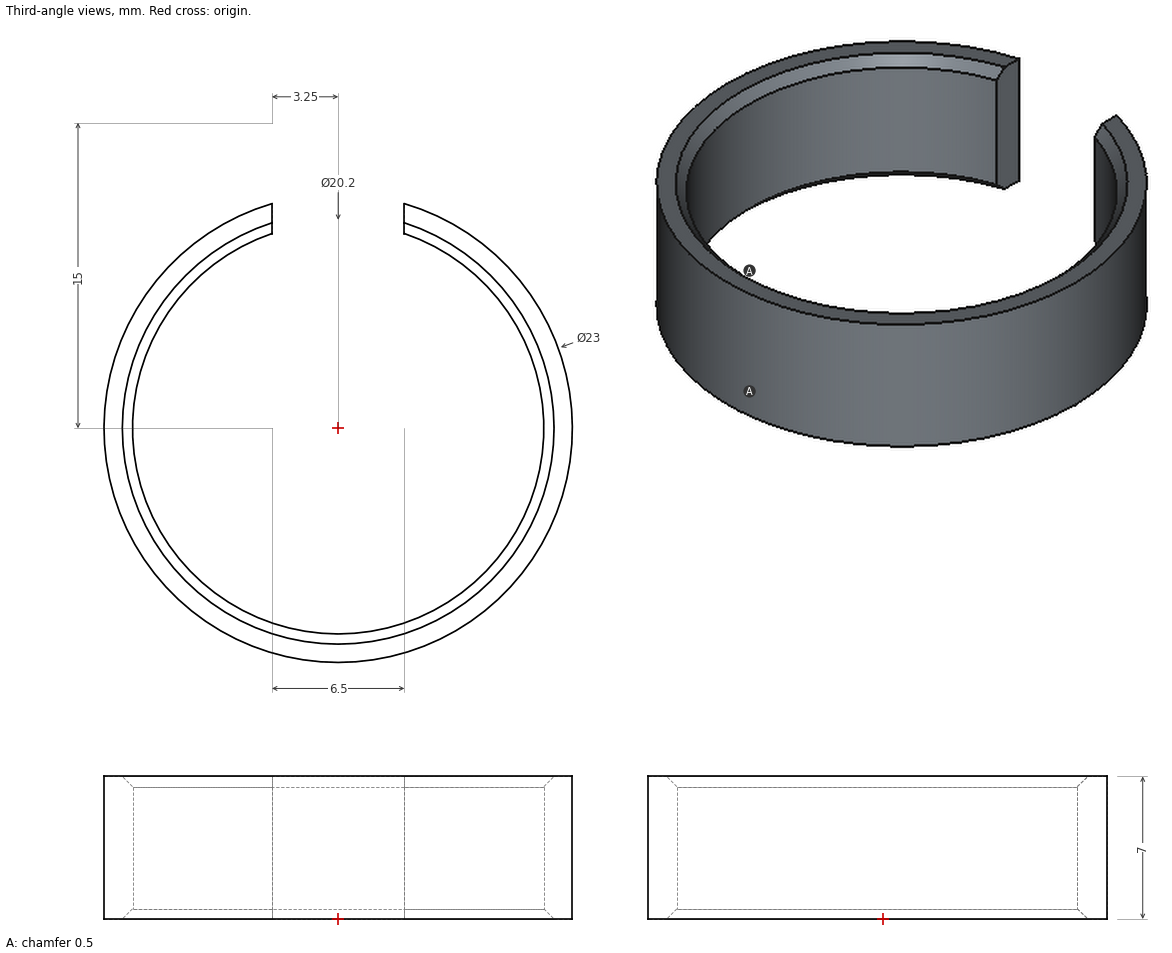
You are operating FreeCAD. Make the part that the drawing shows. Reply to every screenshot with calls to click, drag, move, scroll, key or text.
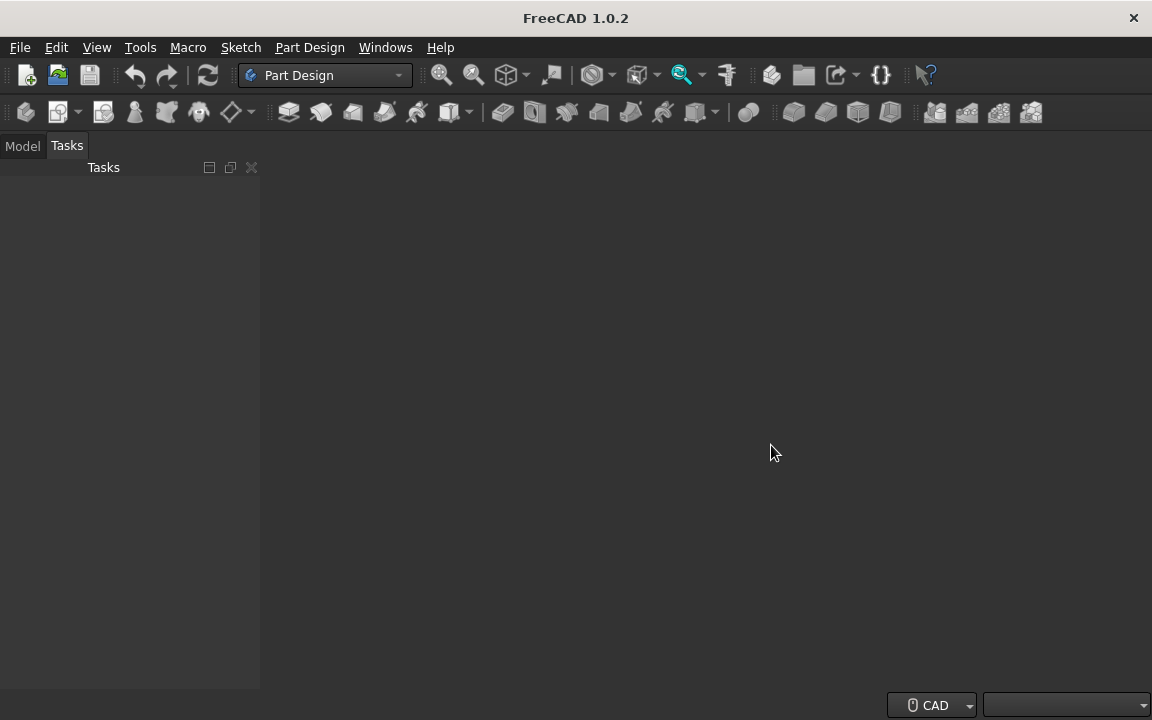
click(26, 76)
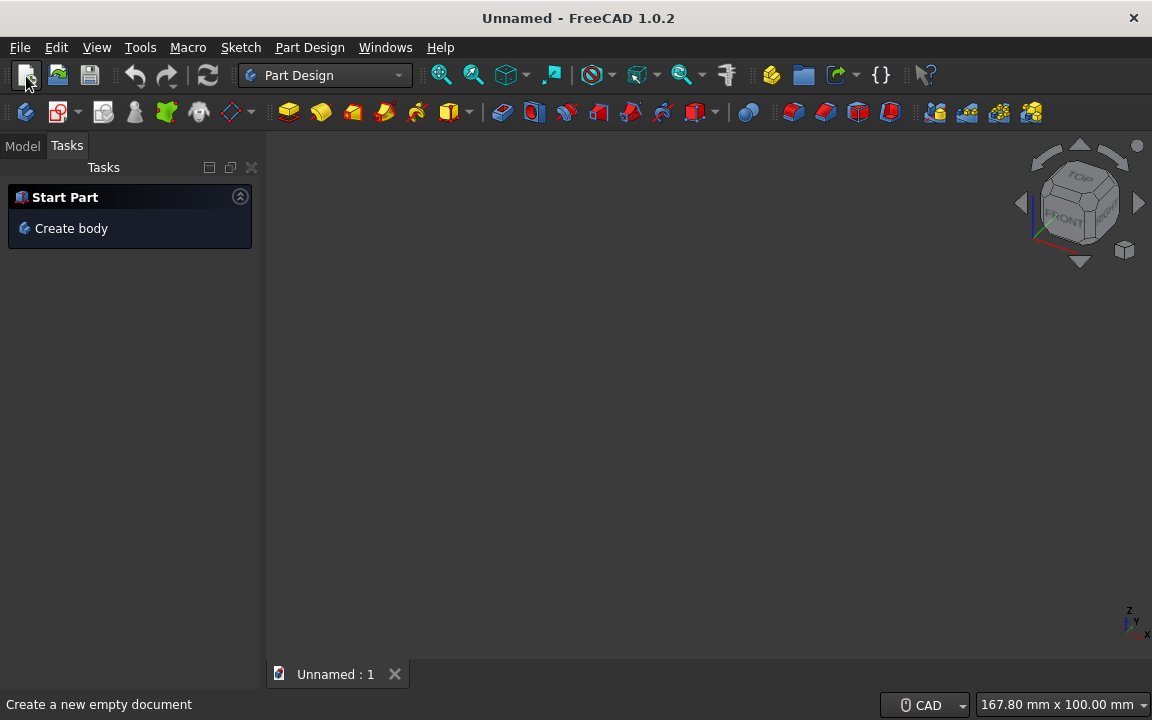
click(58, 112)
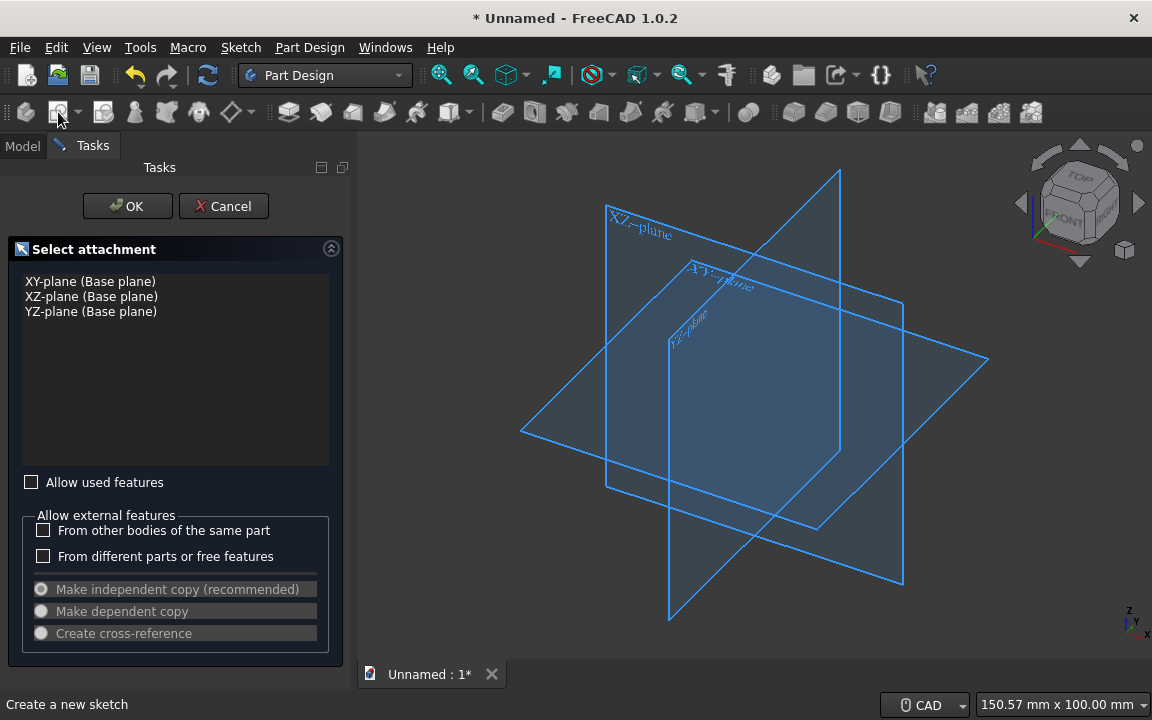
click(82, 282)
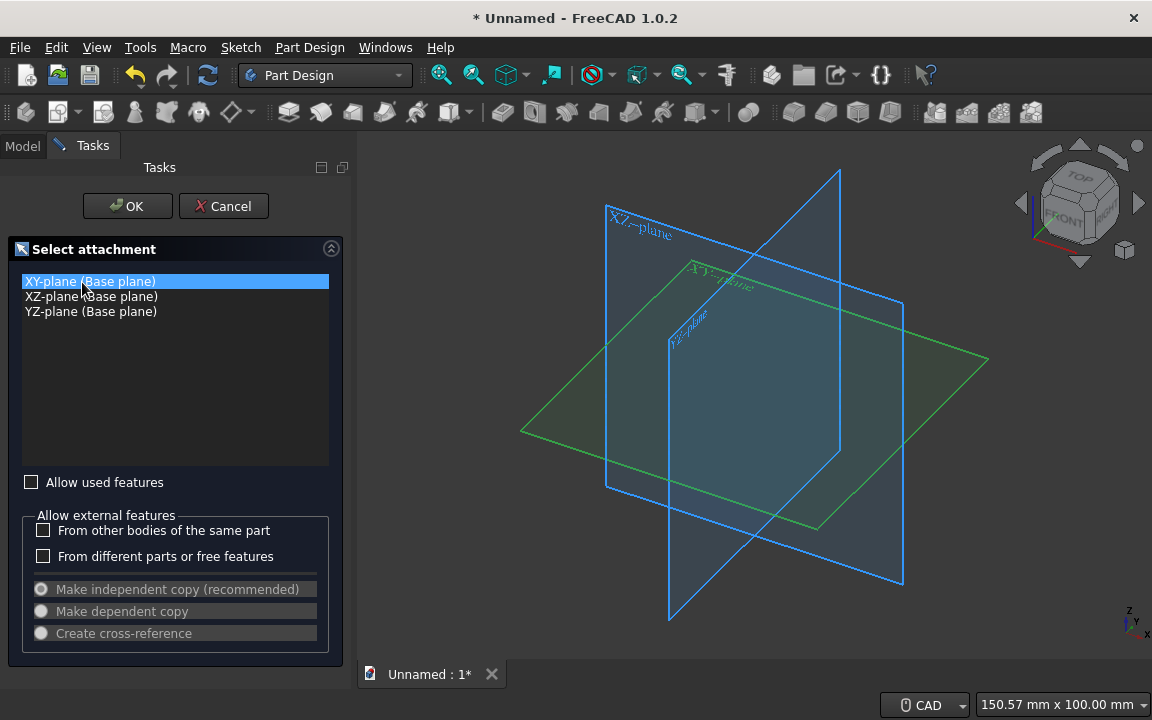
click(128, 206)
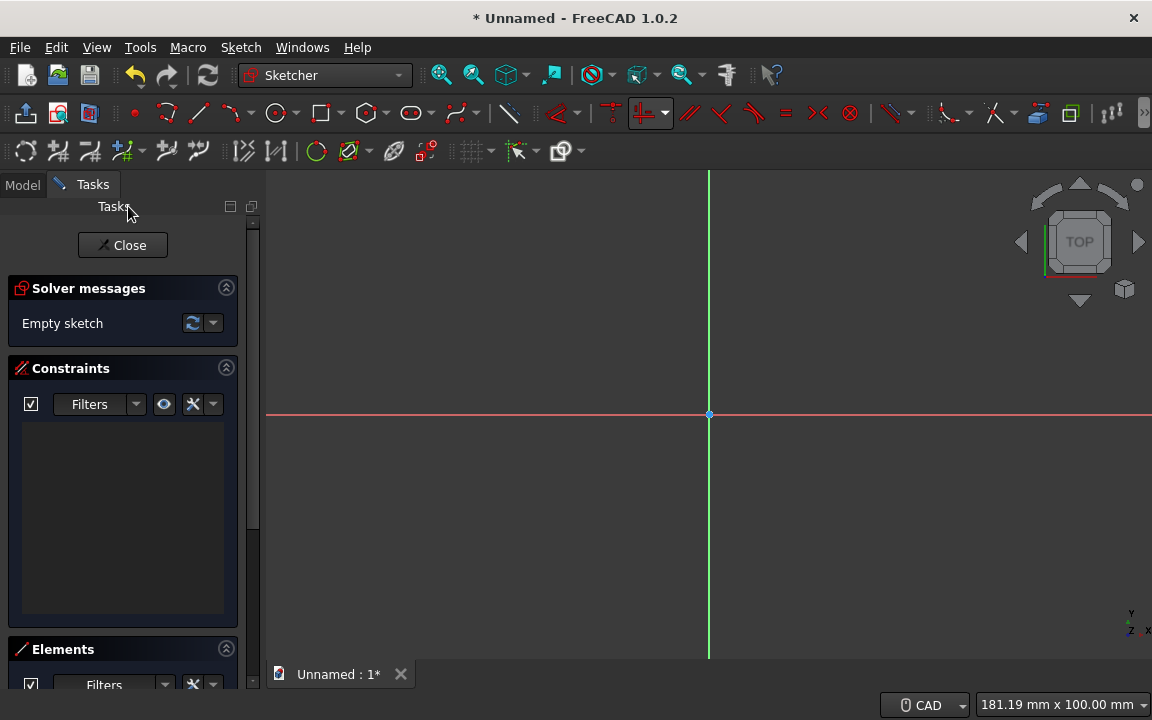
scroll(749, 415, up, 5)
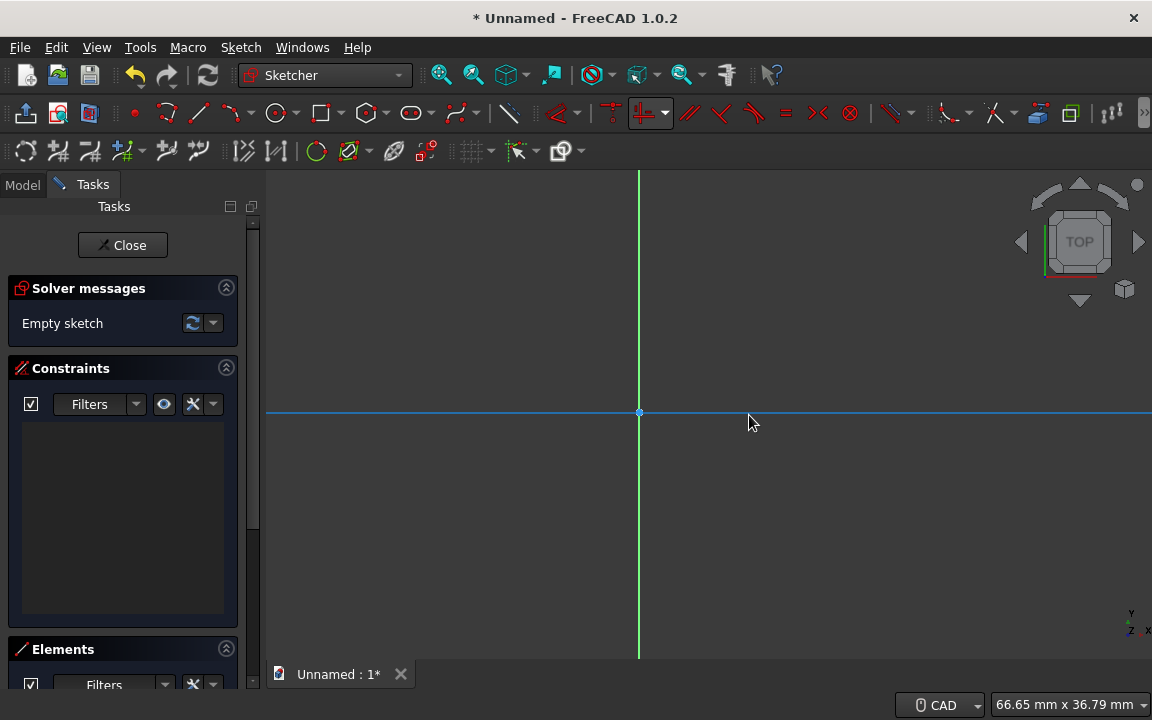
click(276, 114)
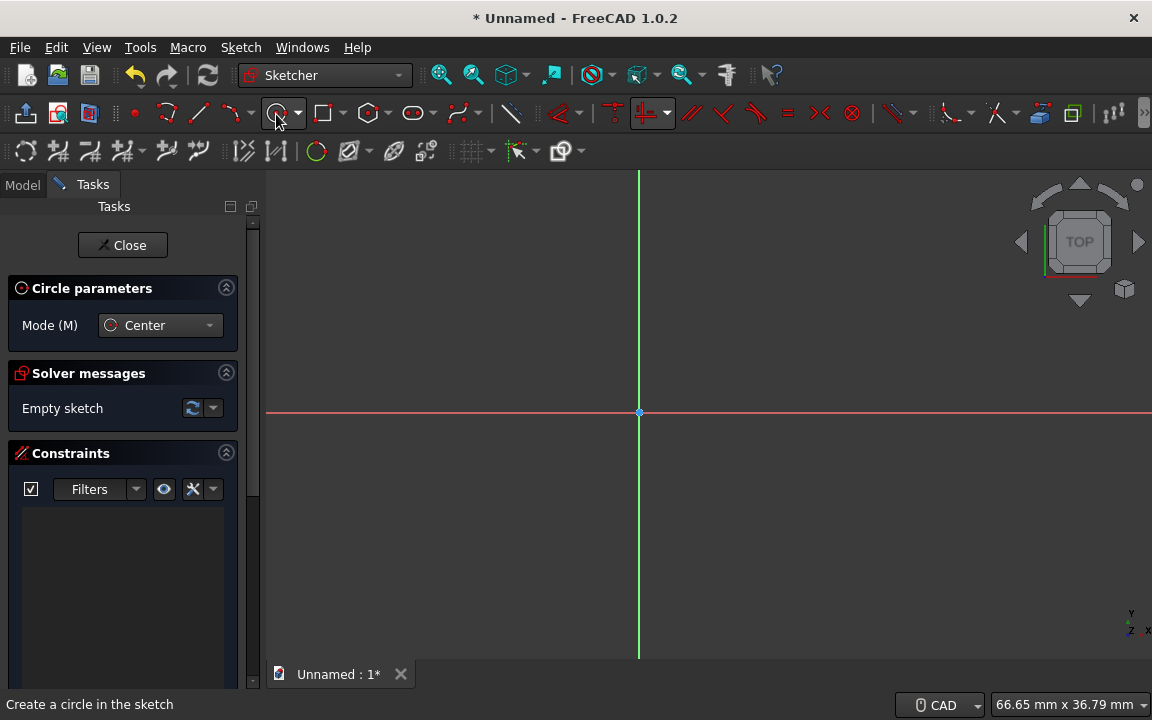
click(639, 413)
click(747, 305)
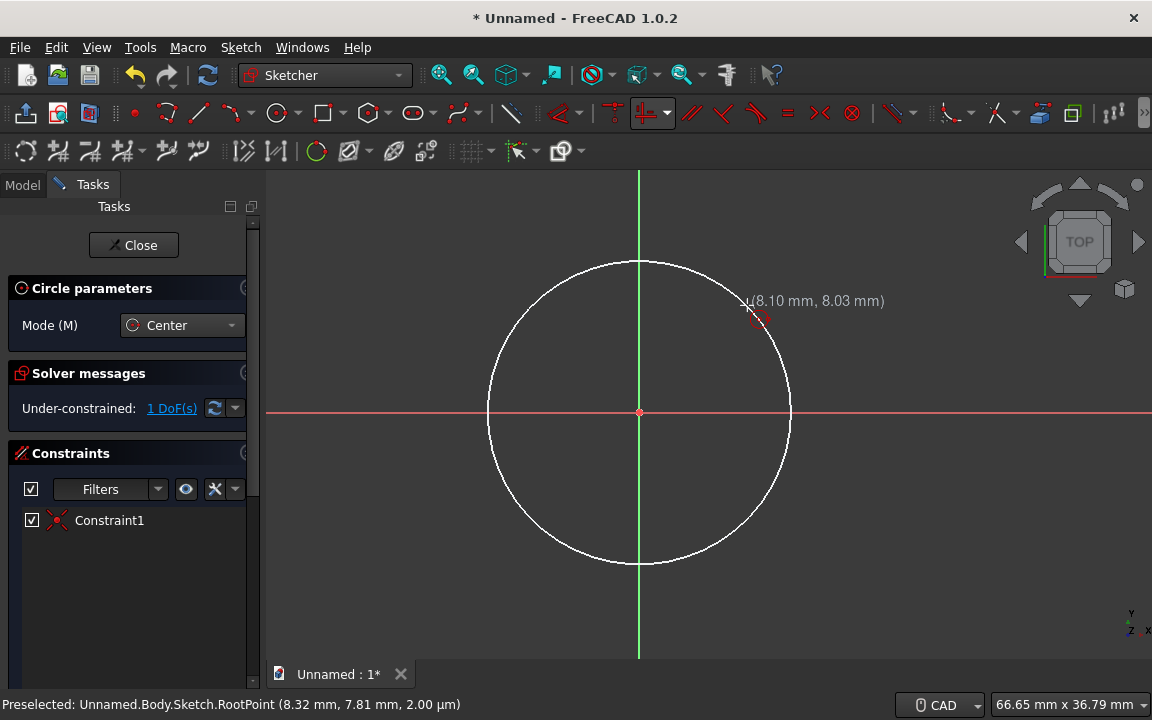
click(639, 413)
click(734, 318)
key(Escape)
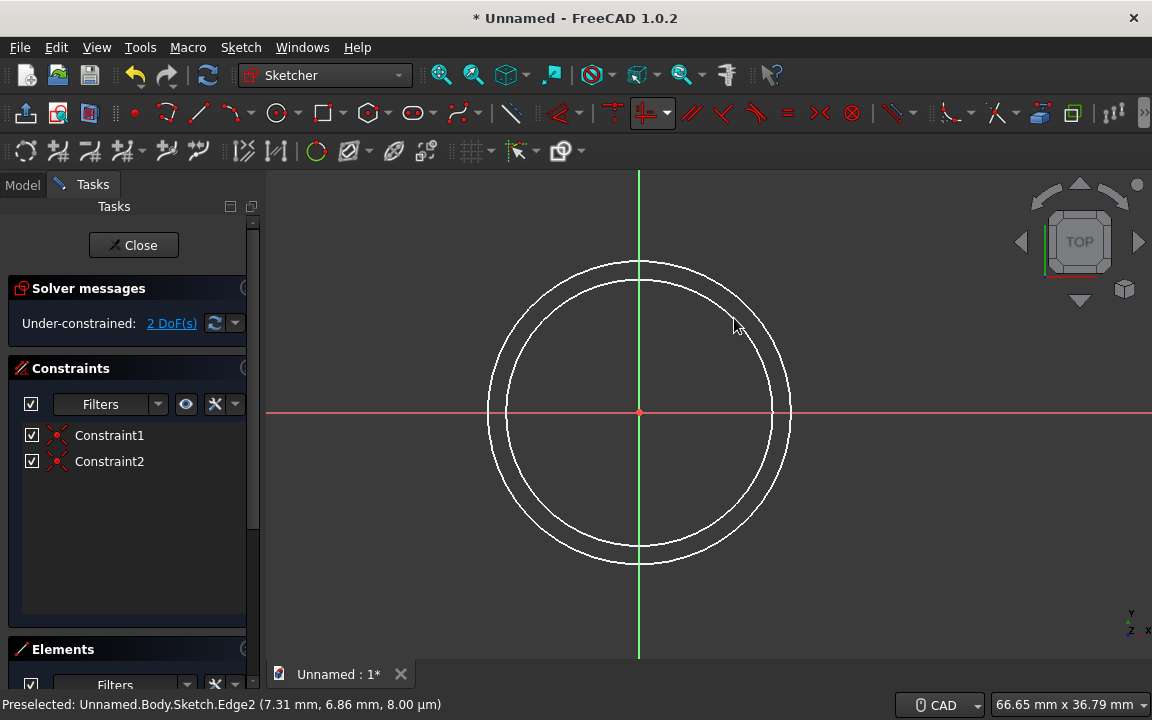
click(558, 114)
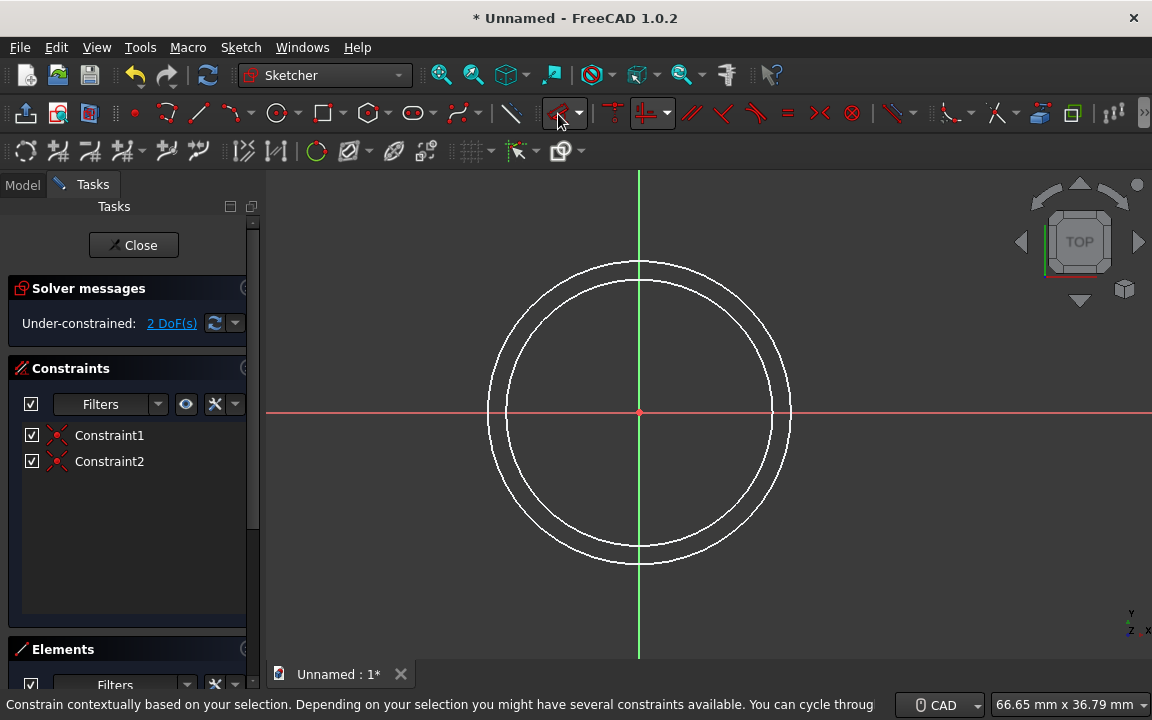
click(746, 305)
click(769, 282)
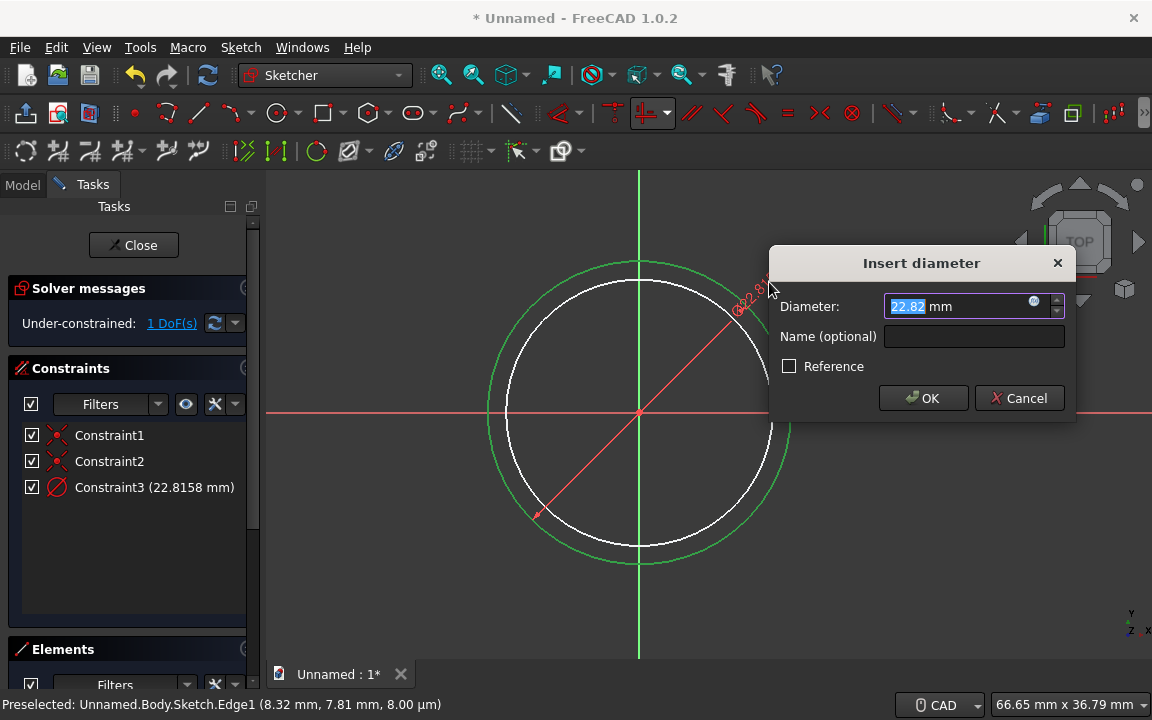
text(23)
key(Return)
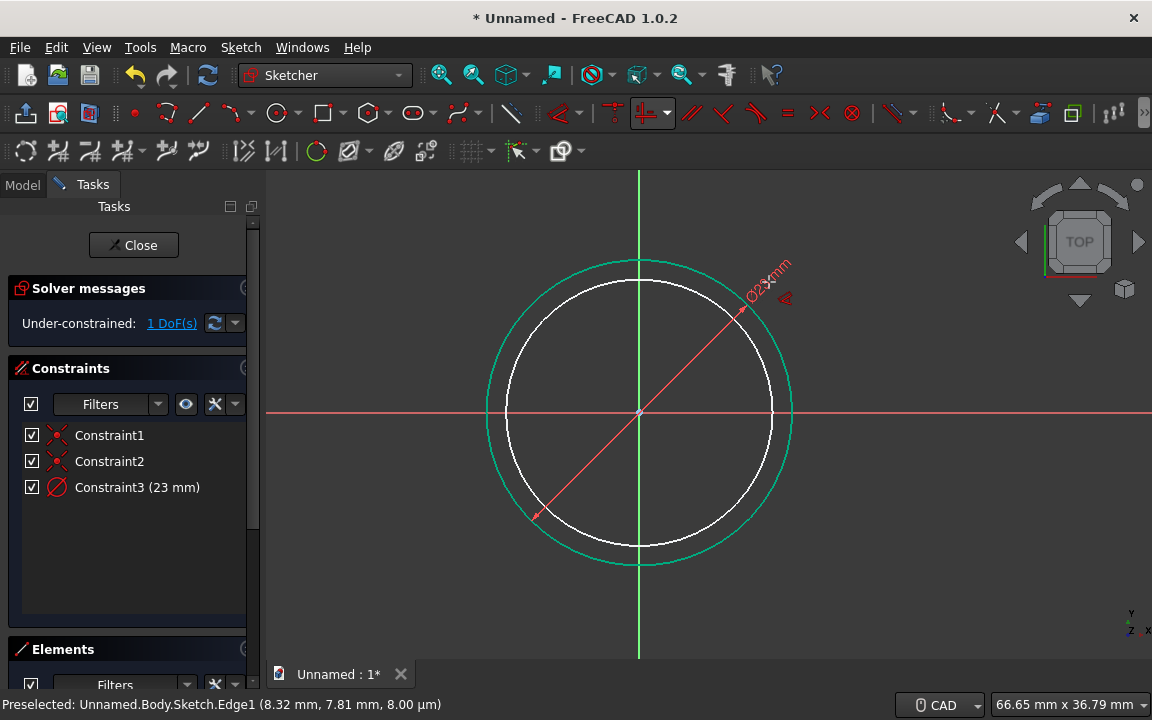
click(733, 318)
click(820, 359)